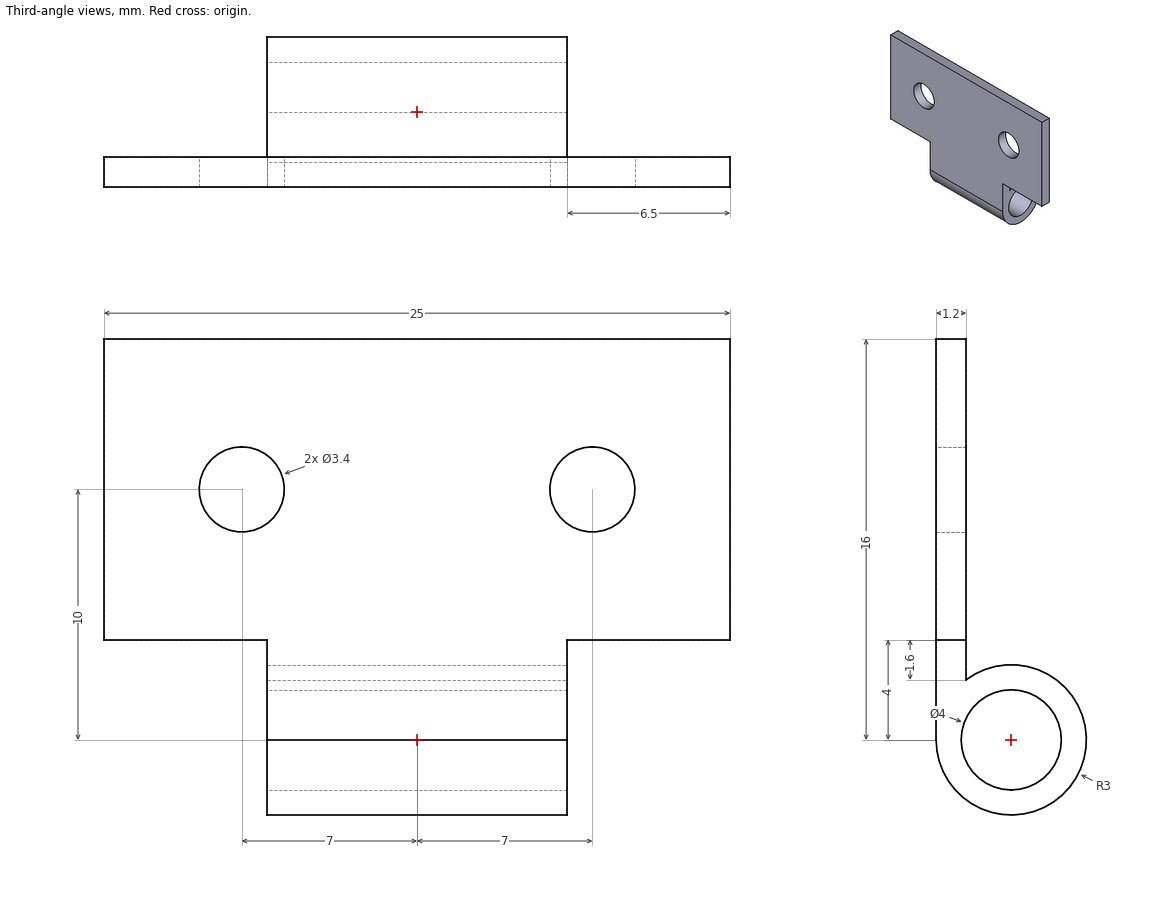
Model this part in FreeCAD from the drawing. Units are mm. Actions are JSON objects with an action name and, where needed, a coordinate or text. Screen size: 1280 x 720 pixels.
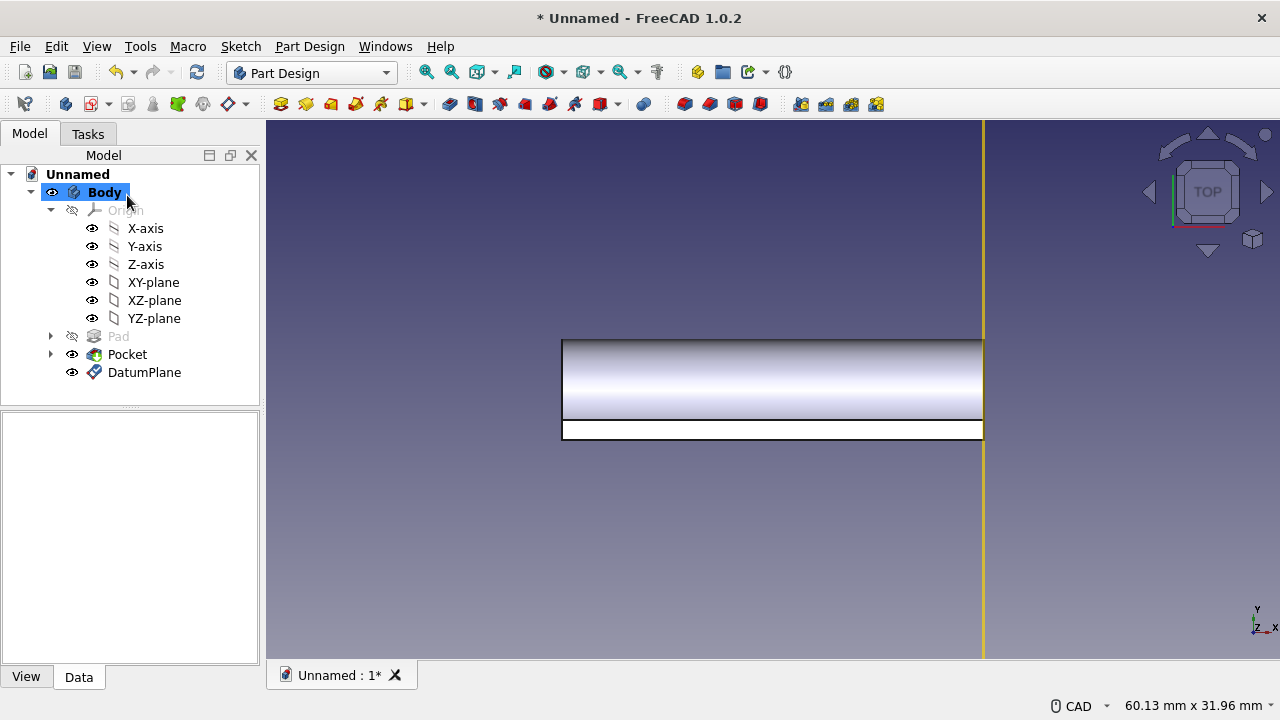
{"action": "left_click", "coordinate": [117, 372]}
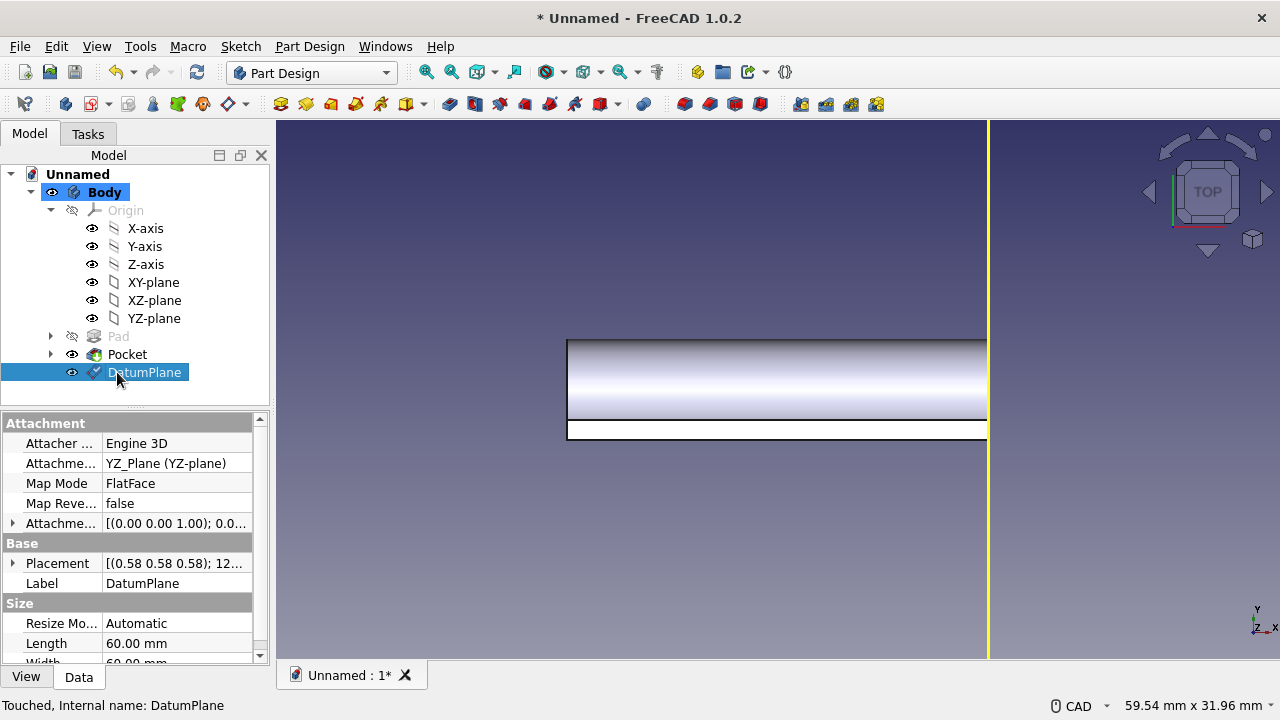
{"action": "left_click", "coordinate": [90, 104]}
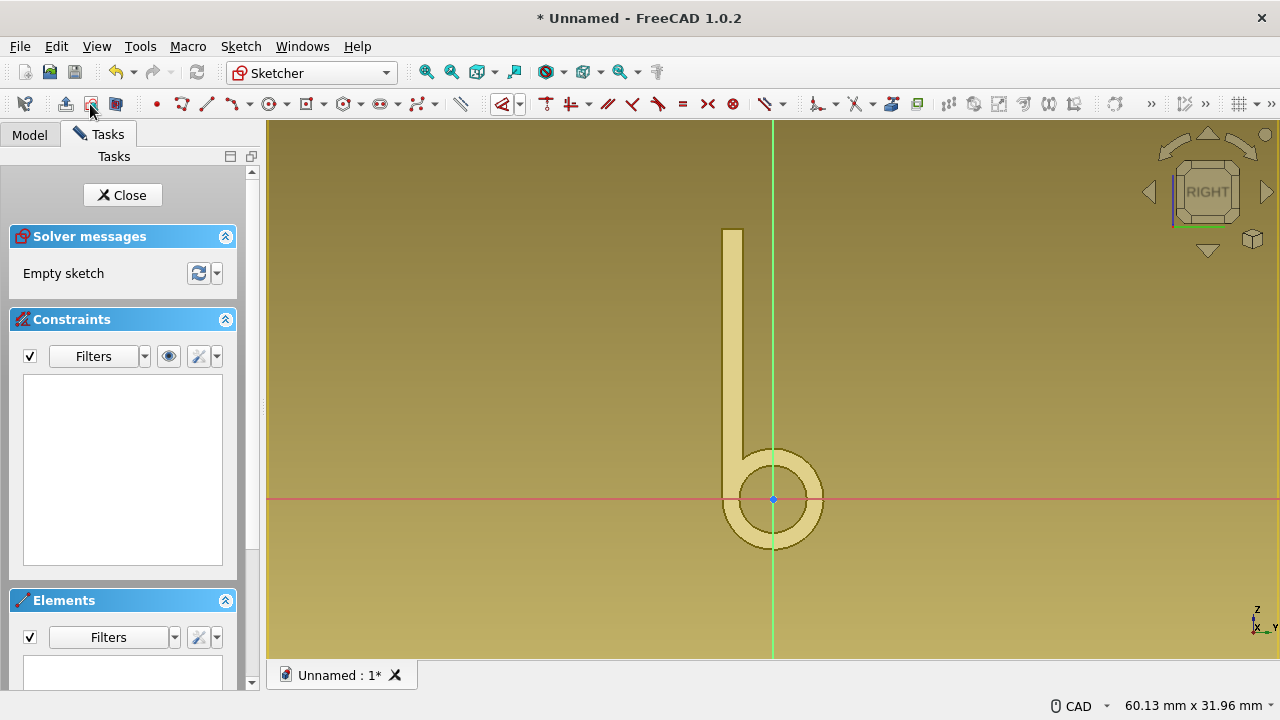
{"action": "scroll", "coordinate": [792, 505], "scroll_direction": "up", "scroll_amount": 7}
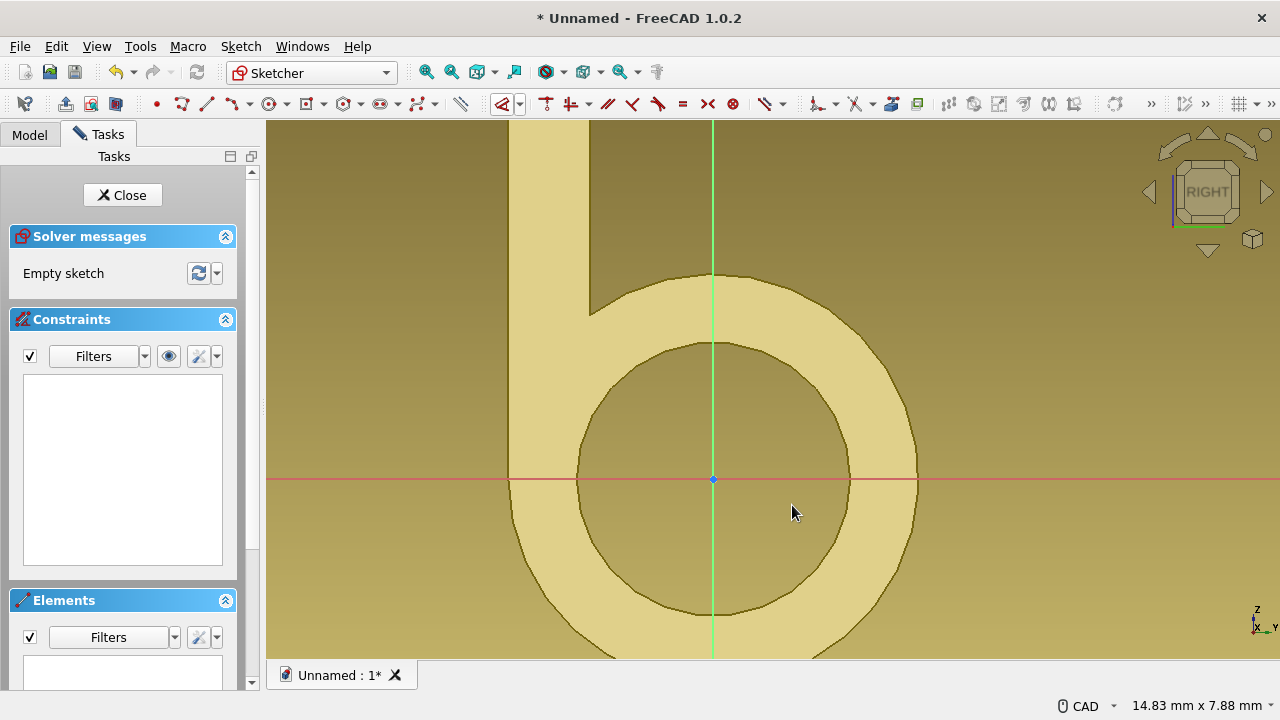
{"action": "left_click", "coordinate": [182, 104]}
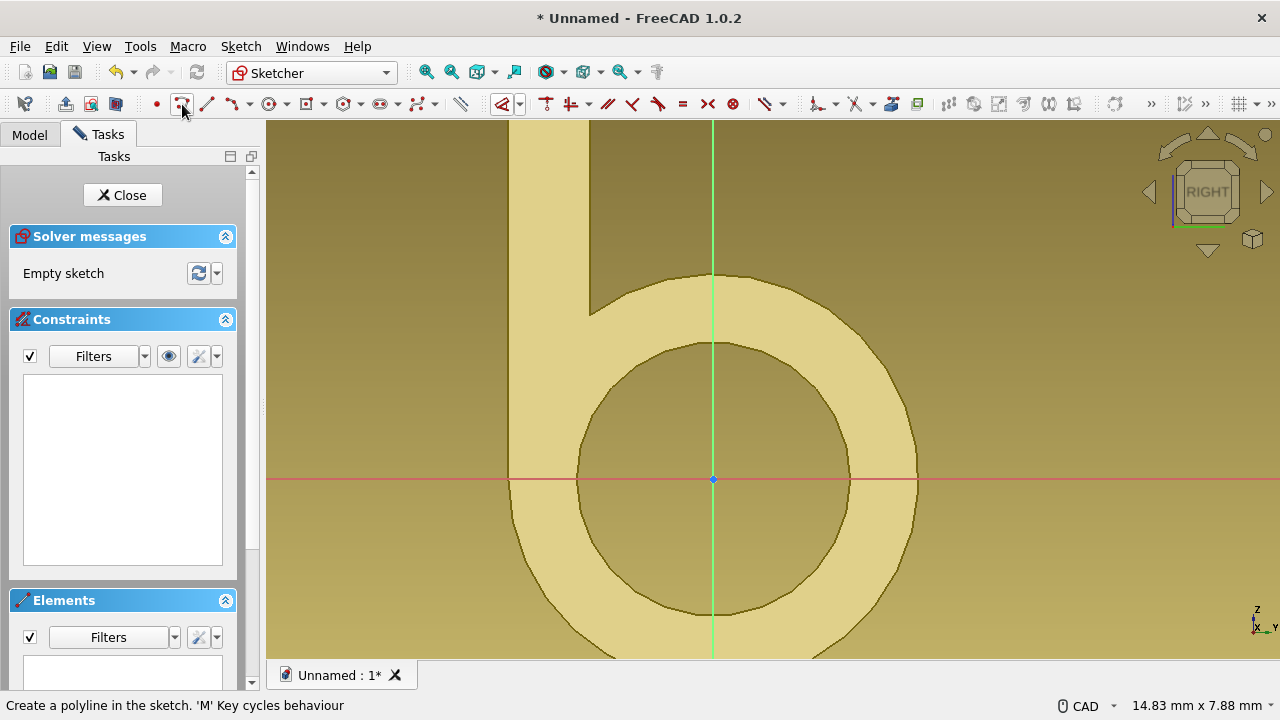
{"action": "left_click", "coordinate": [590, 315]}
{"action": "left_click", "coordinate": [590, 206]}
{"action": "left_click", "coordinate": [508, 206]}
{"action": "left_click", "coordinate": [508, 479]}
{"action": "right_click", "coordinate": [508, 479]}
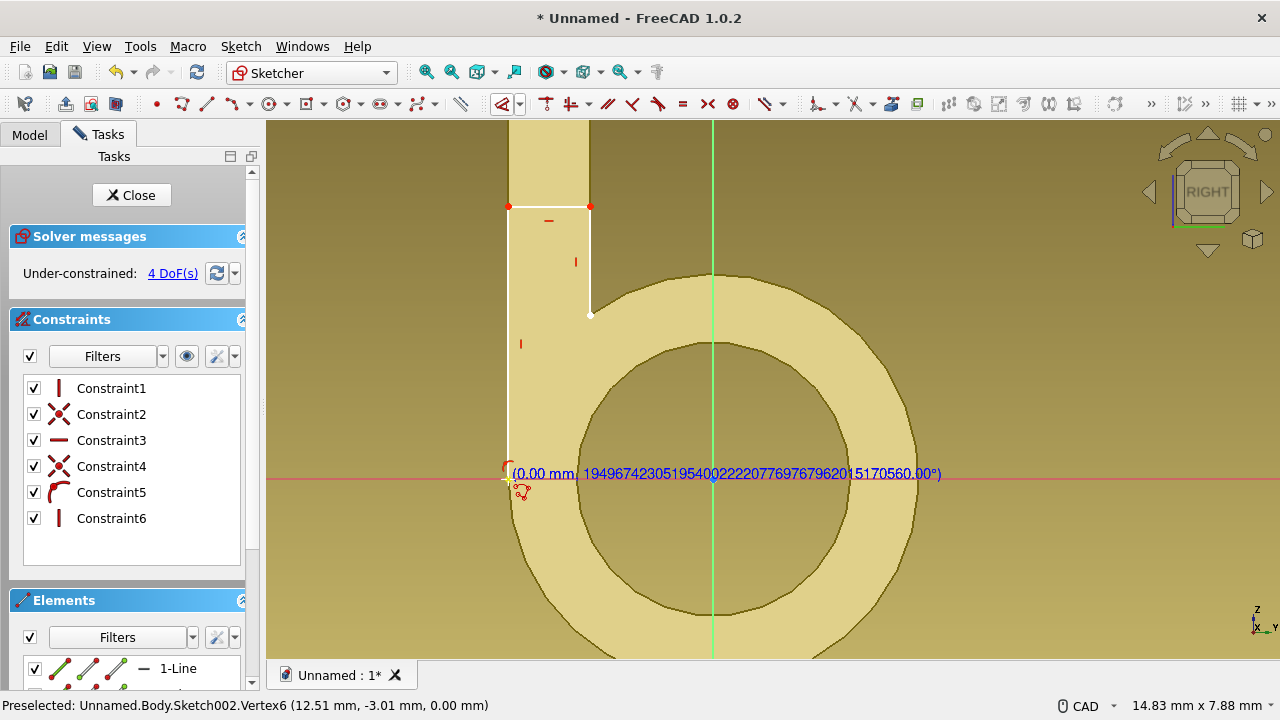
{"action": "left_click", "coordinate": [232, 104]}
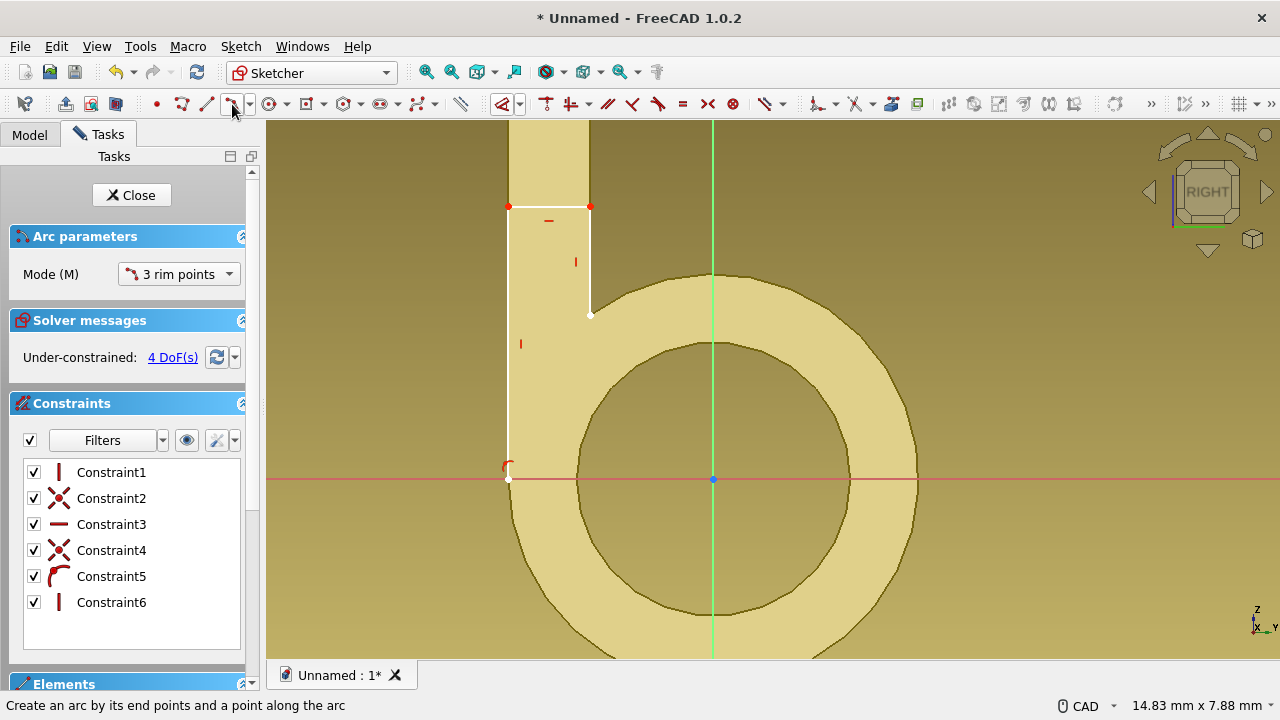
{"action": "left_click", "coordinate": [508, 479]}
{"action": "left_click", "coordinate": [590, 316]}
{"action": "left_click", "coordinate": [897, 571]}
{"action": "key", "text": "Escape"}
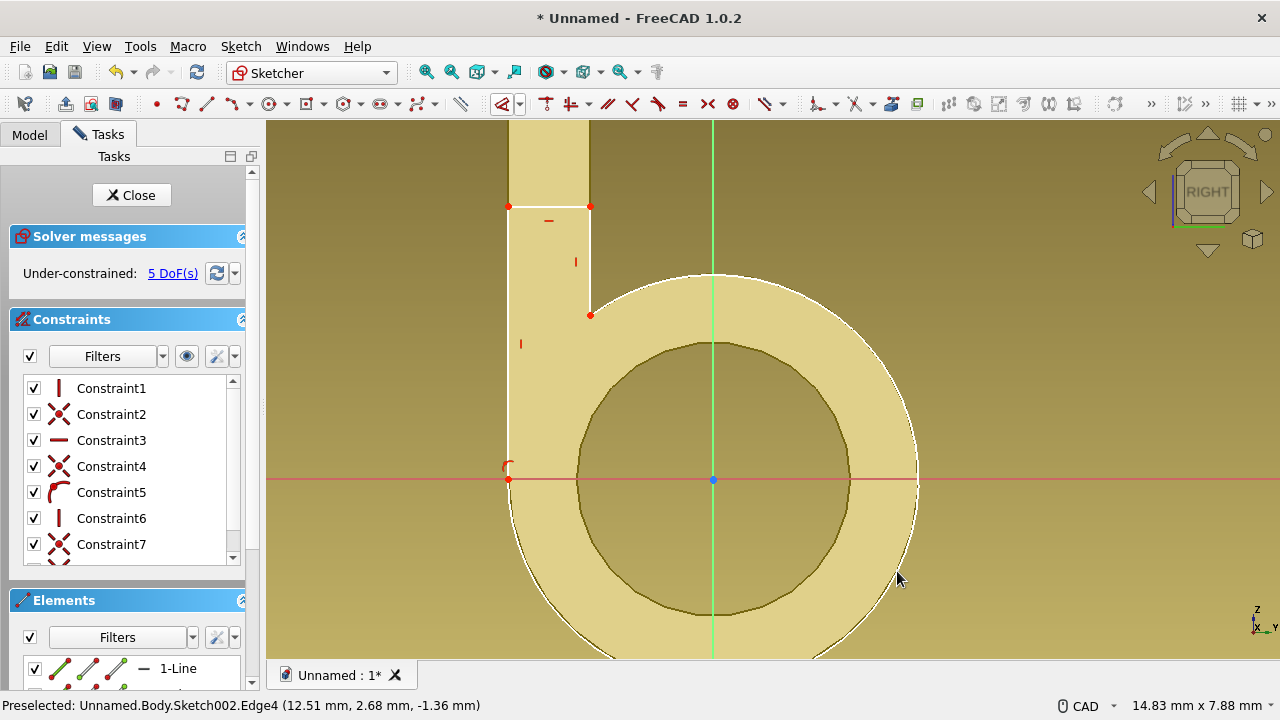
{"action": "left_click", "coordinate": [508, 289]}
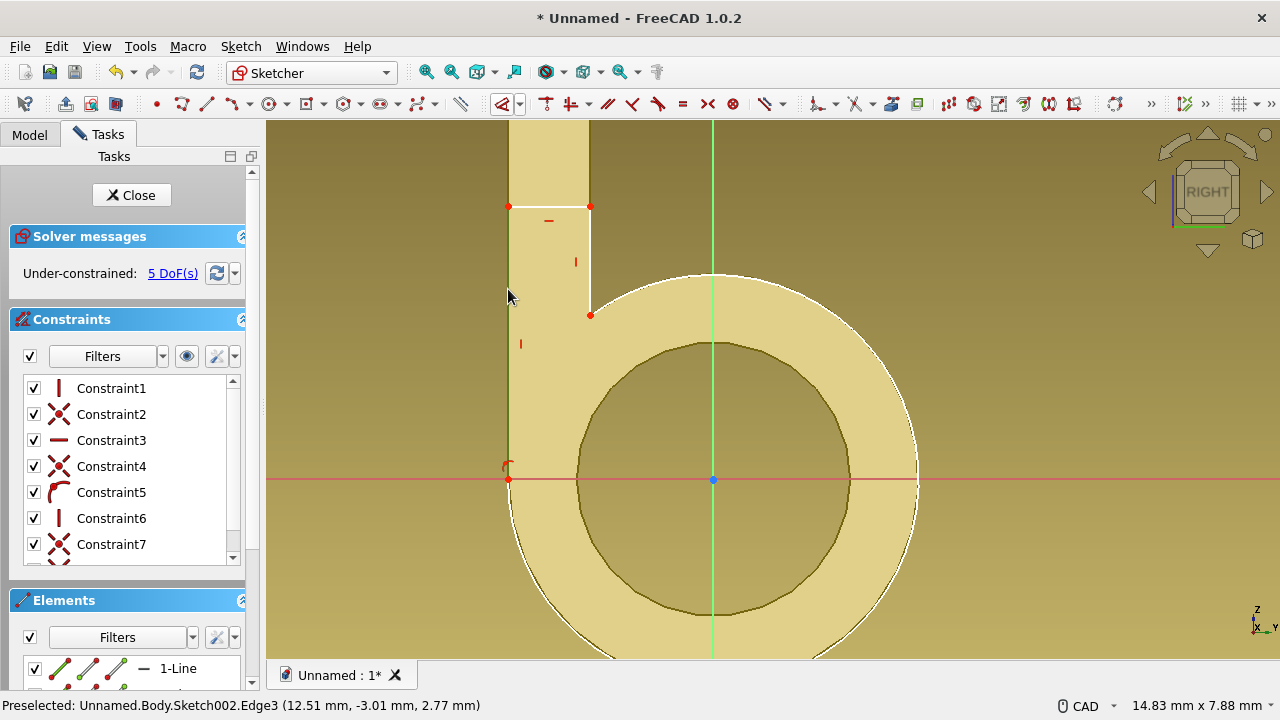
{"action": "left_click", "coordinate": [882, 363]}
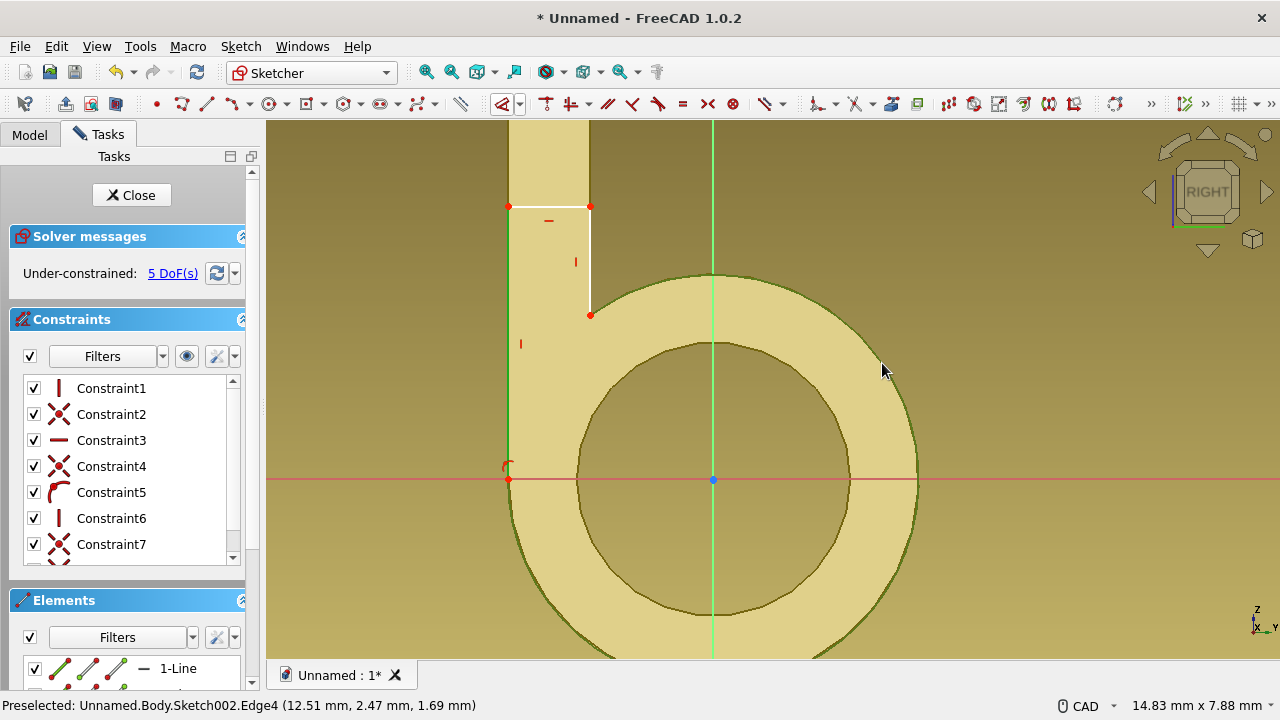
{"action": "left_click", "coordinate": [658, 104]}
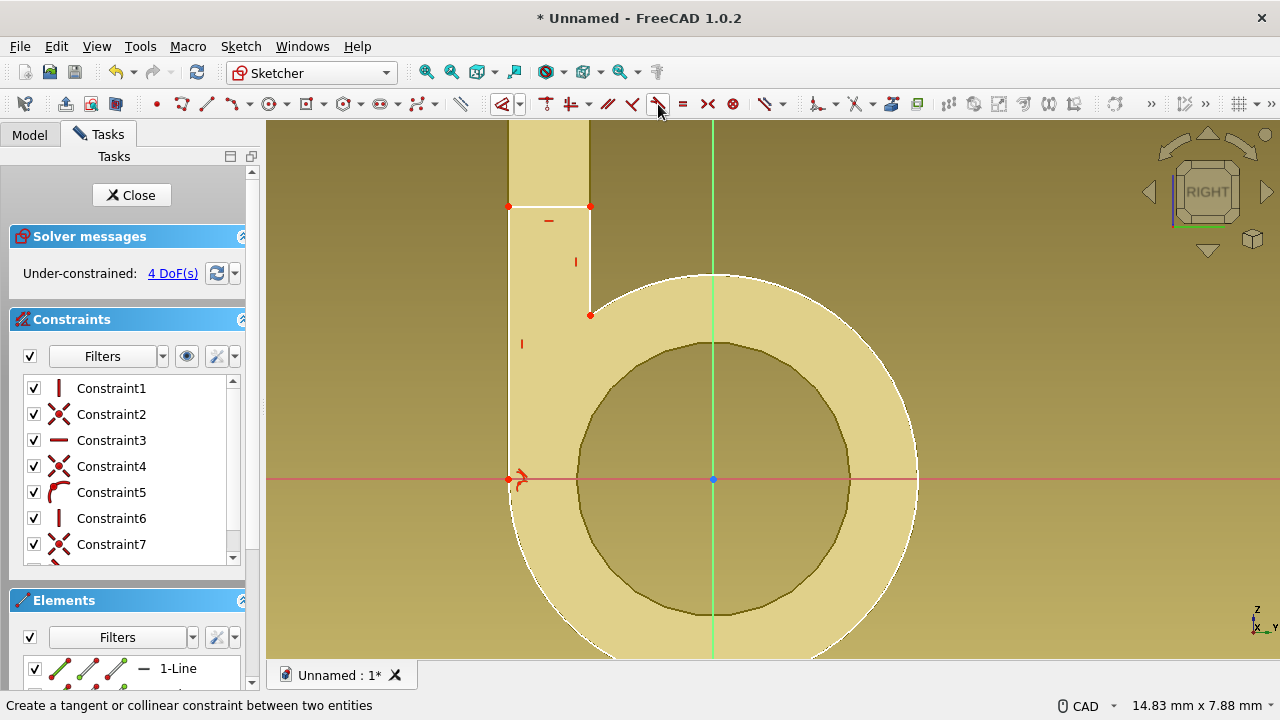
{"action": "left_click", "coordinate": [713, 479]}